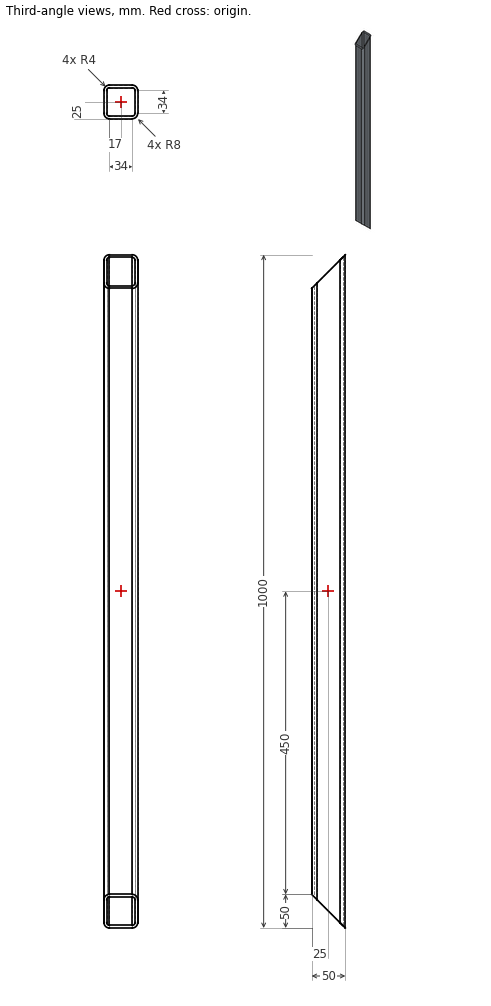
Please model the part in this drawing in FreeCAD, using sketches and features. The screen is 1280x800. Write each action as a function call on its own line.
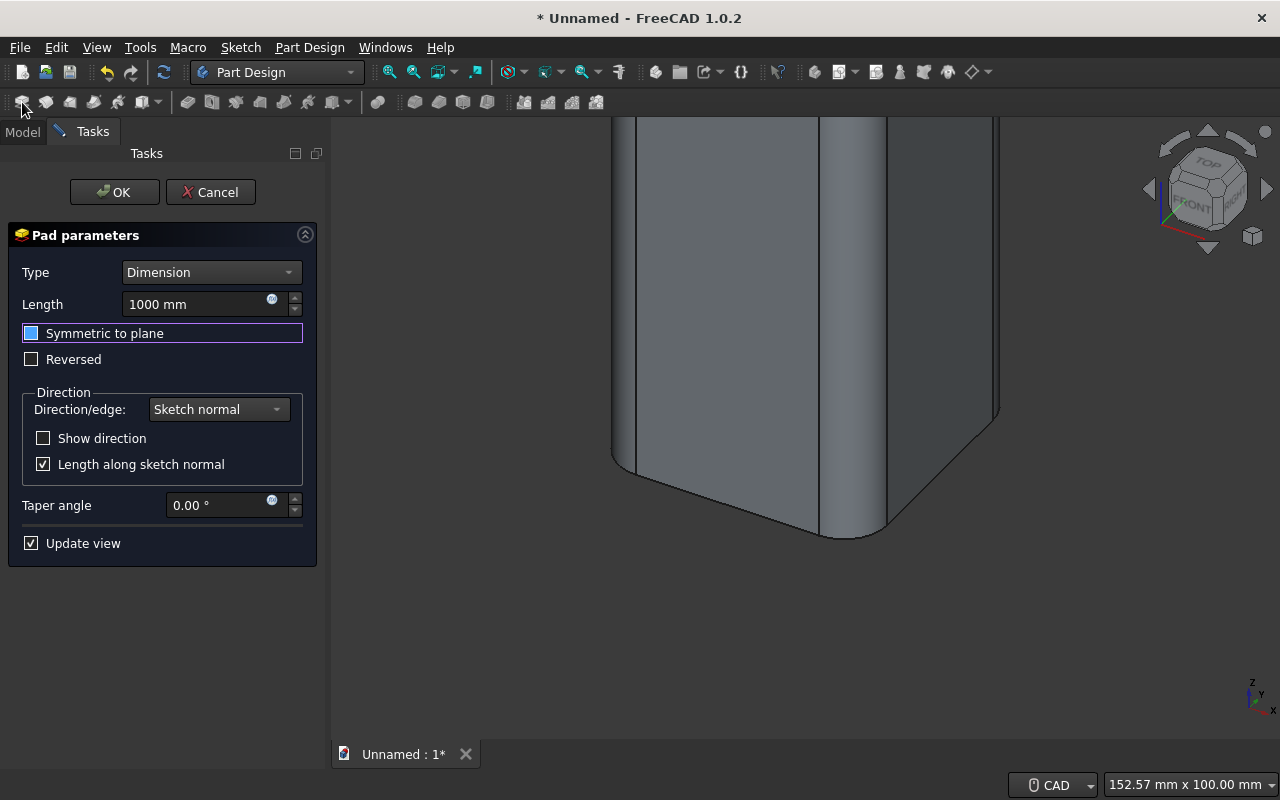
click(30, 333)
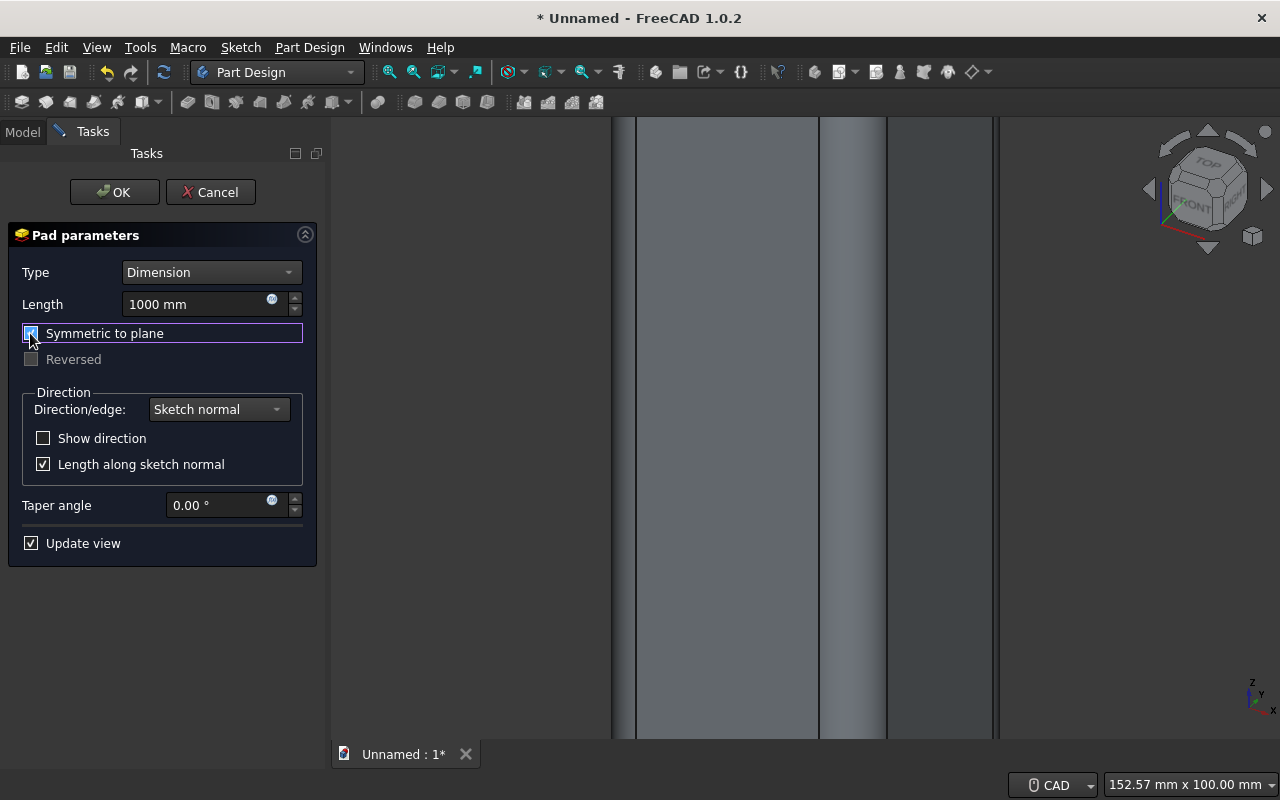
click(115, 192)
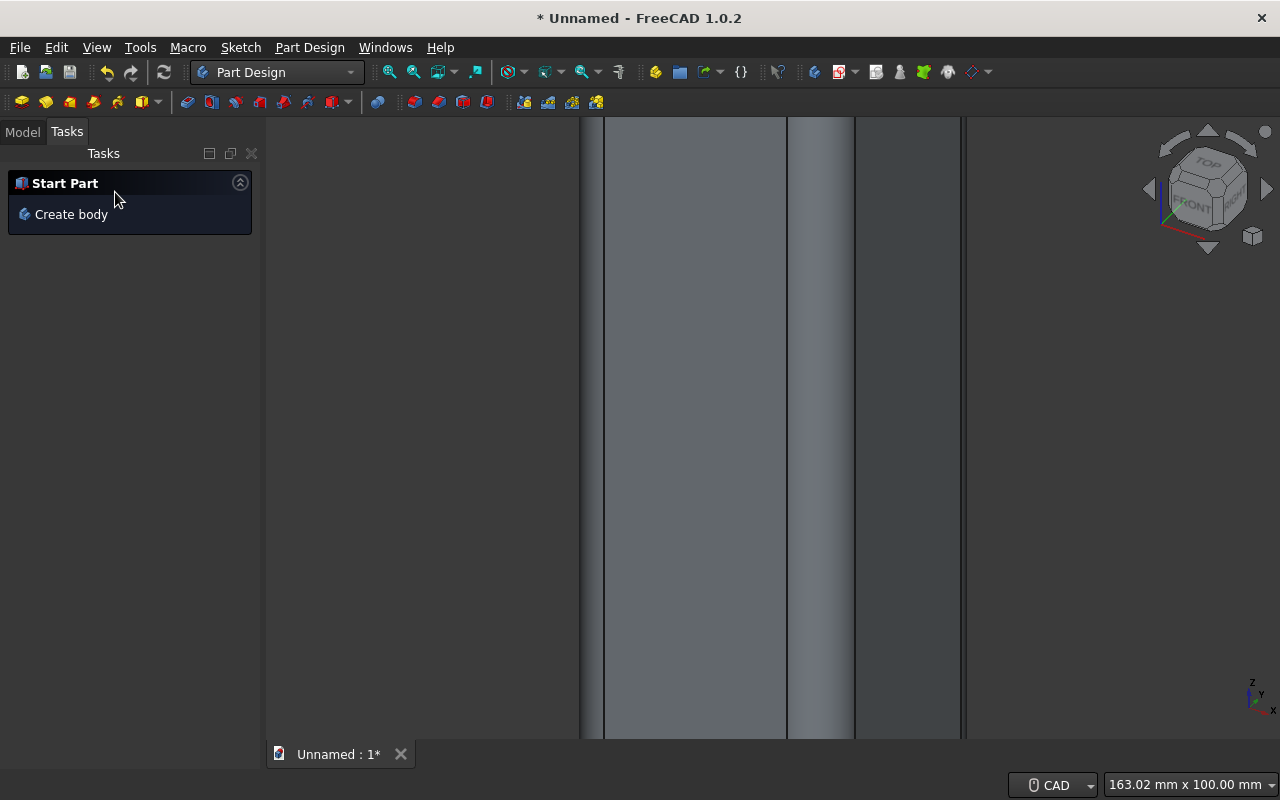
click(390, 72)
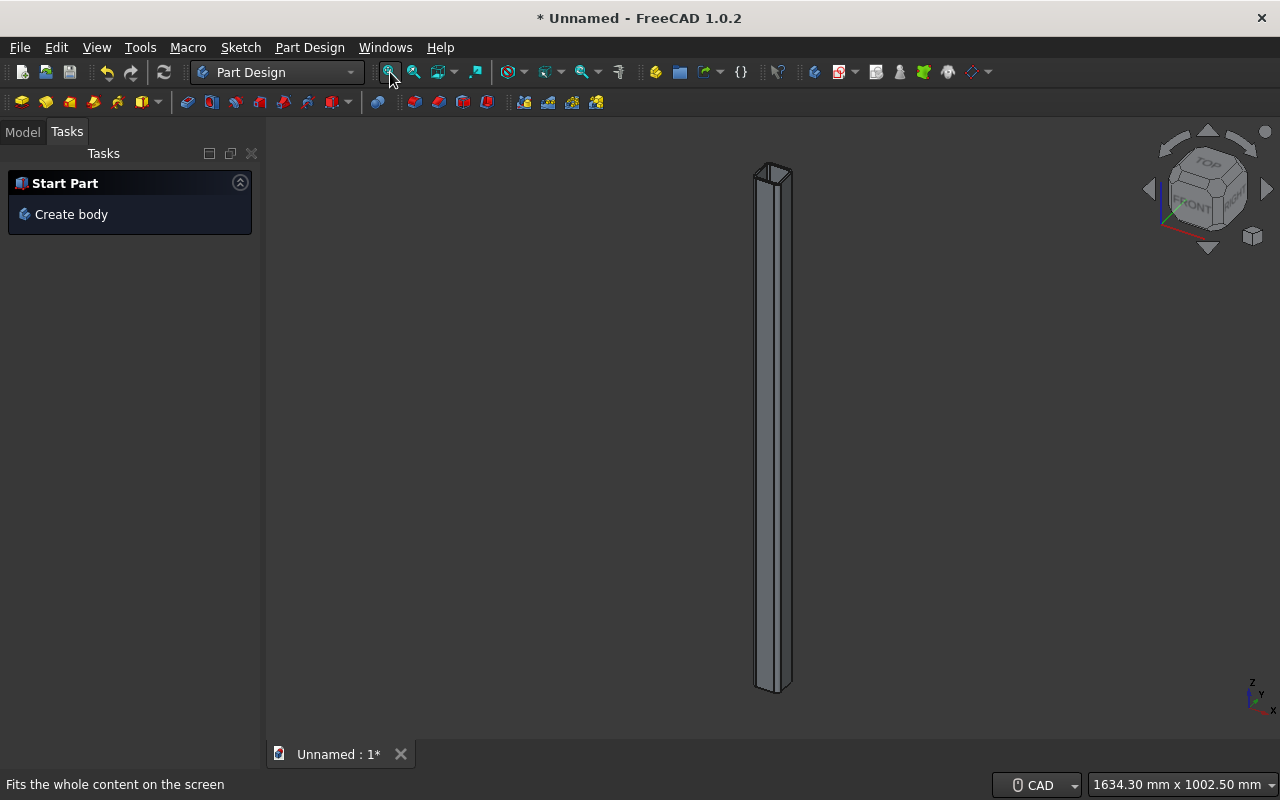
key(6)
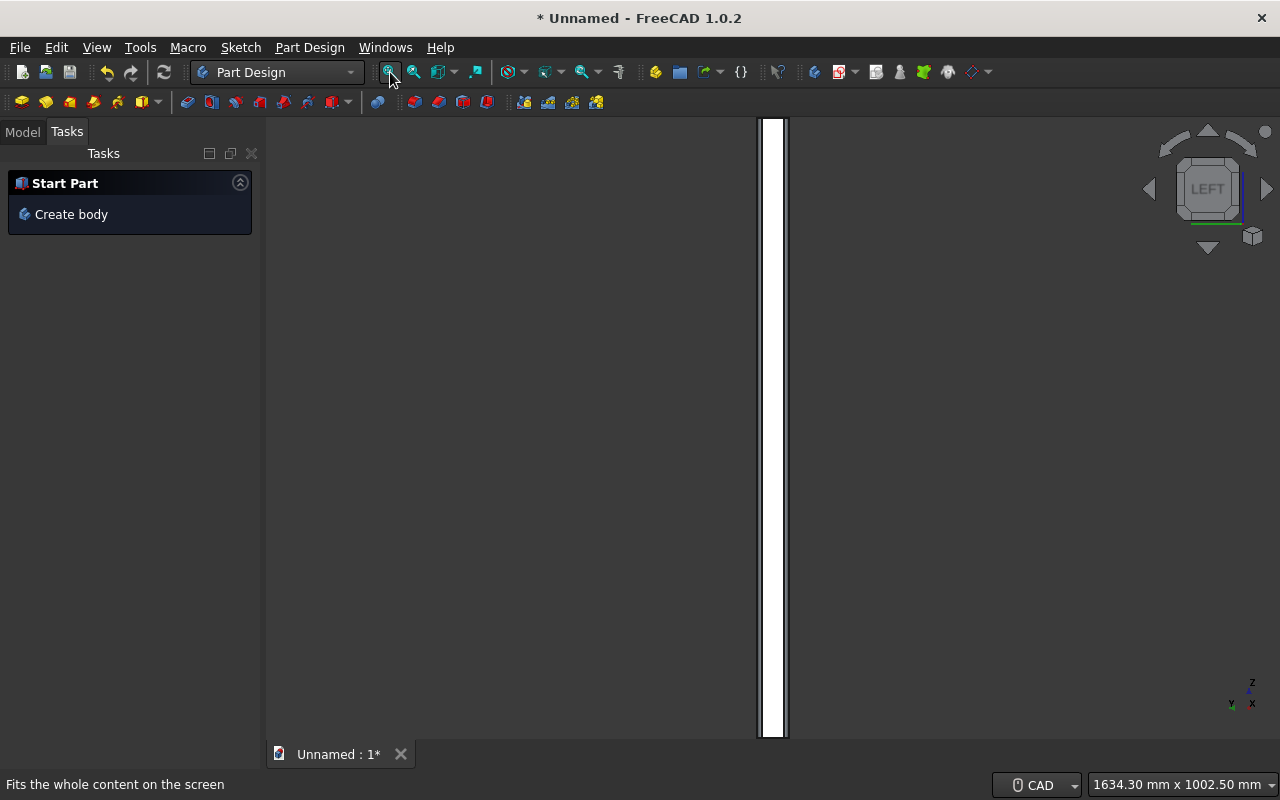
click(773, 161)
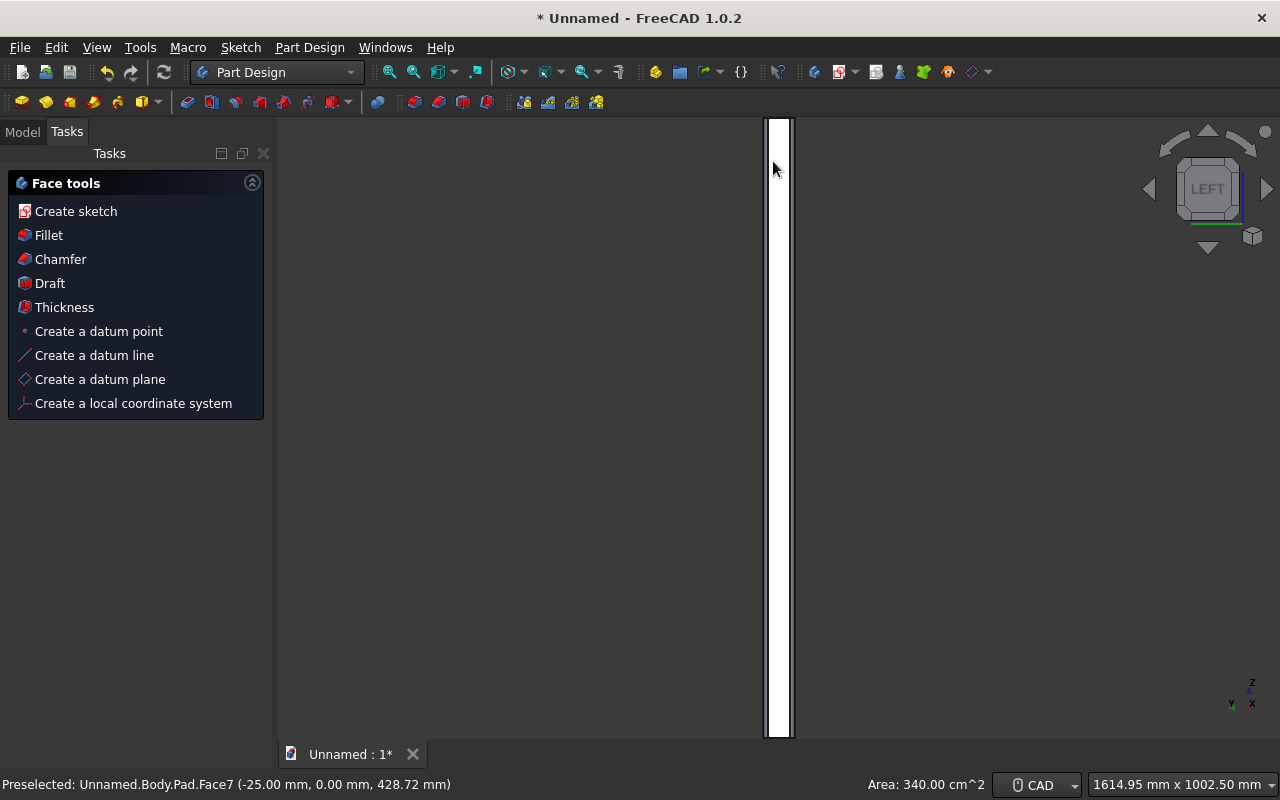
click(840, 72)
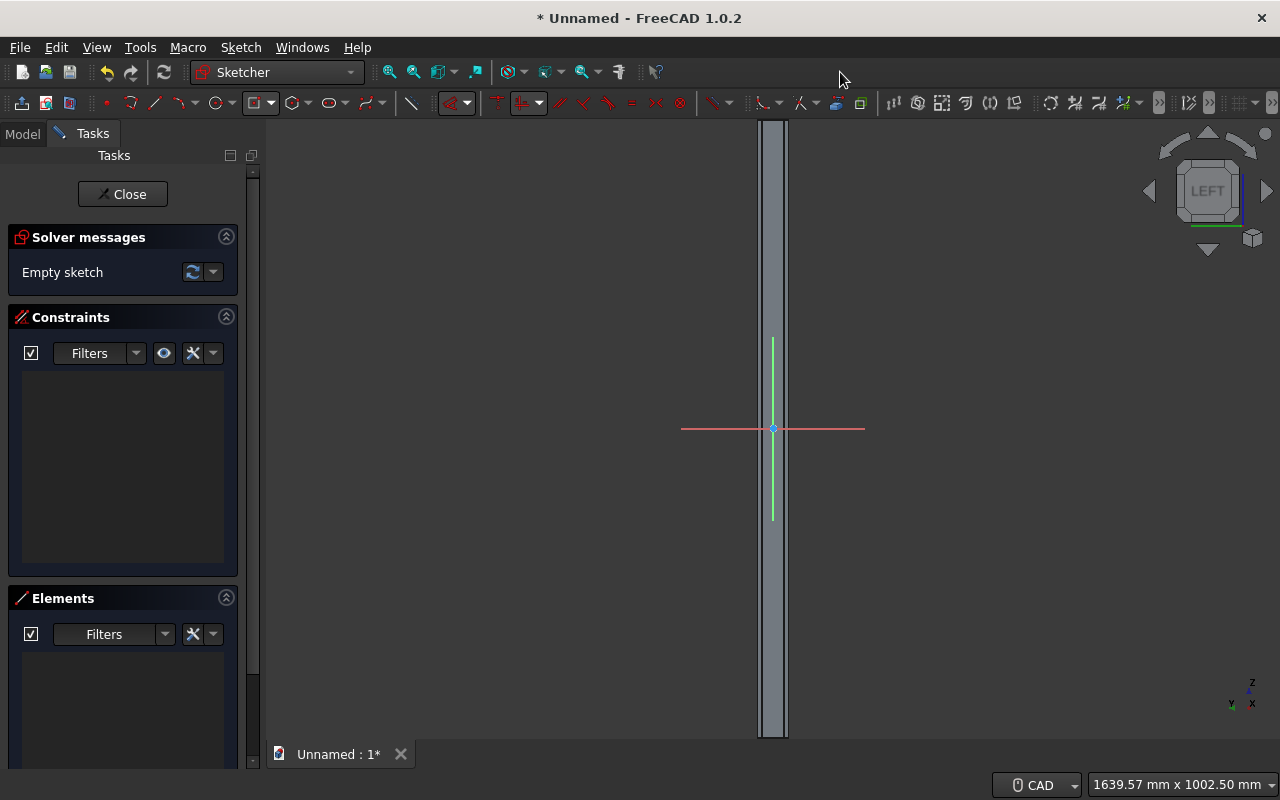
scroll(704, 429, down, 5)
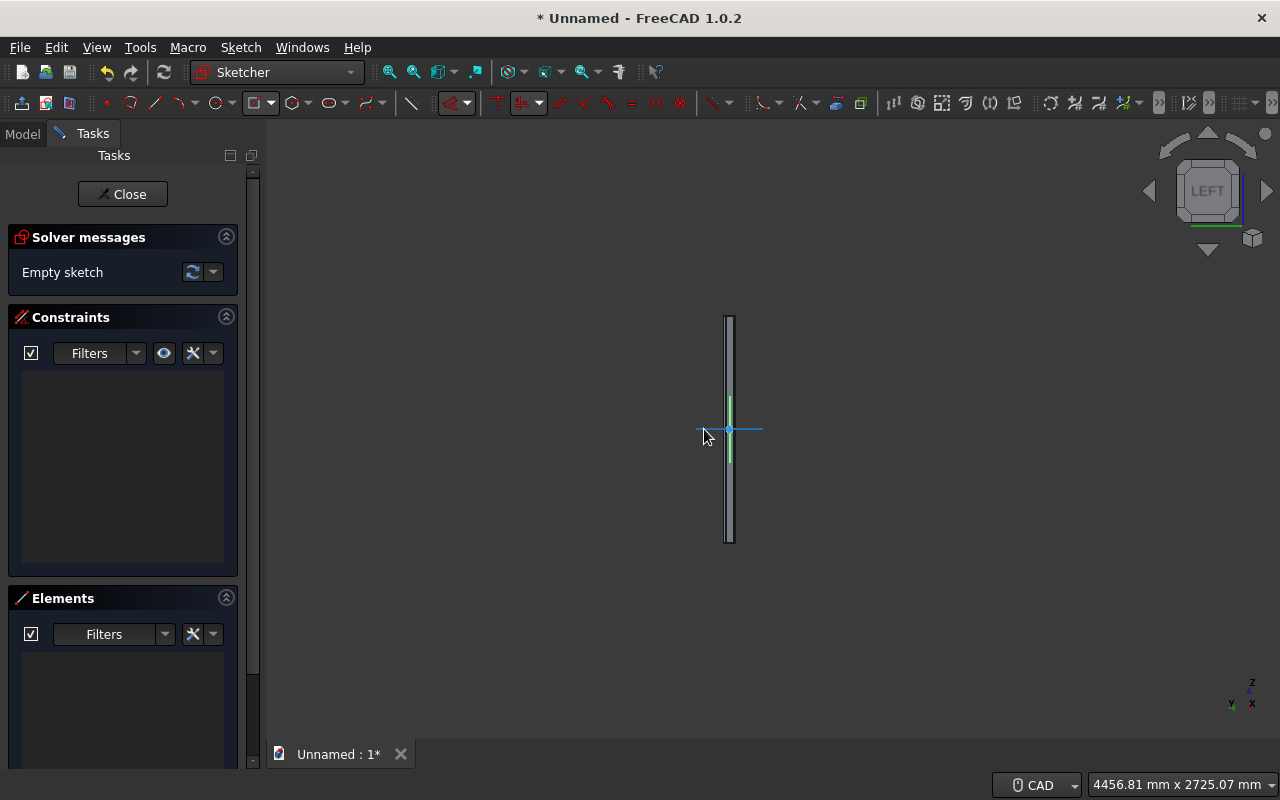
scroll(731, 543, up, 15)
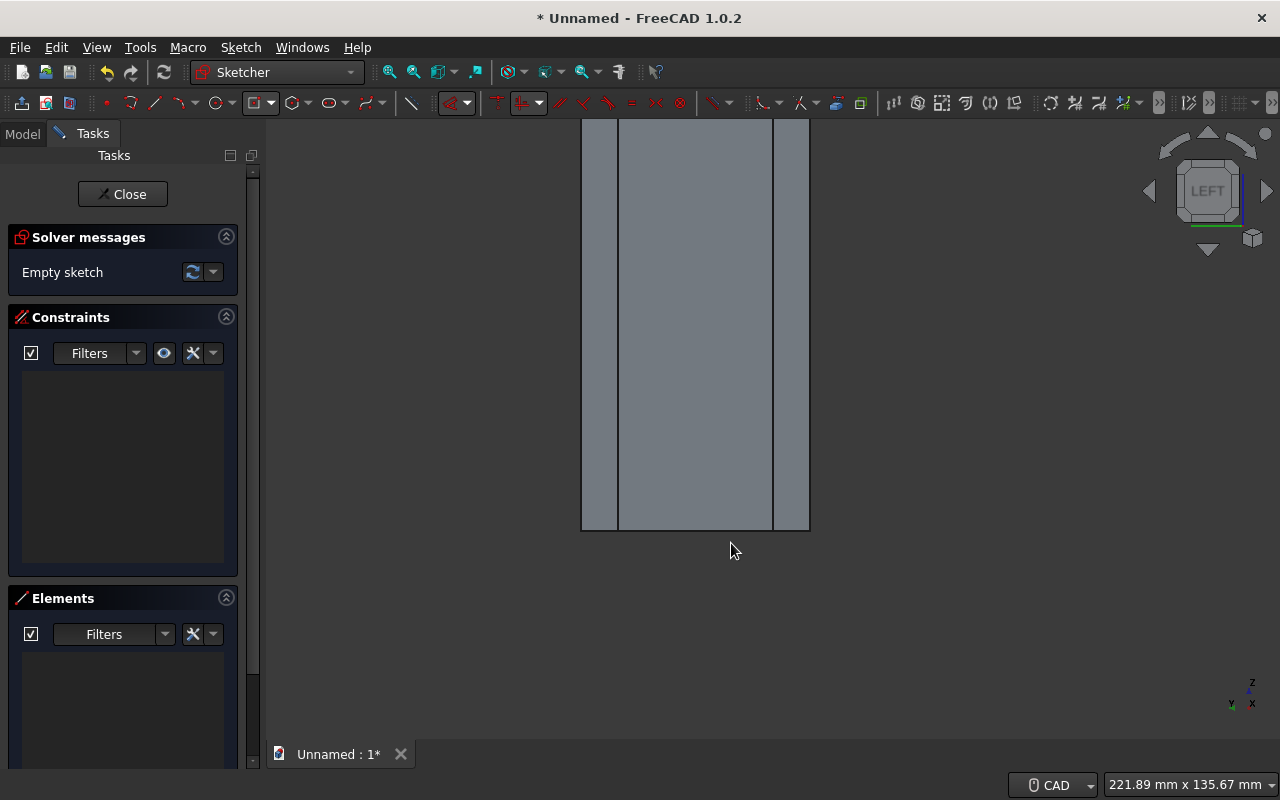
scroll(684, 403, up, 3)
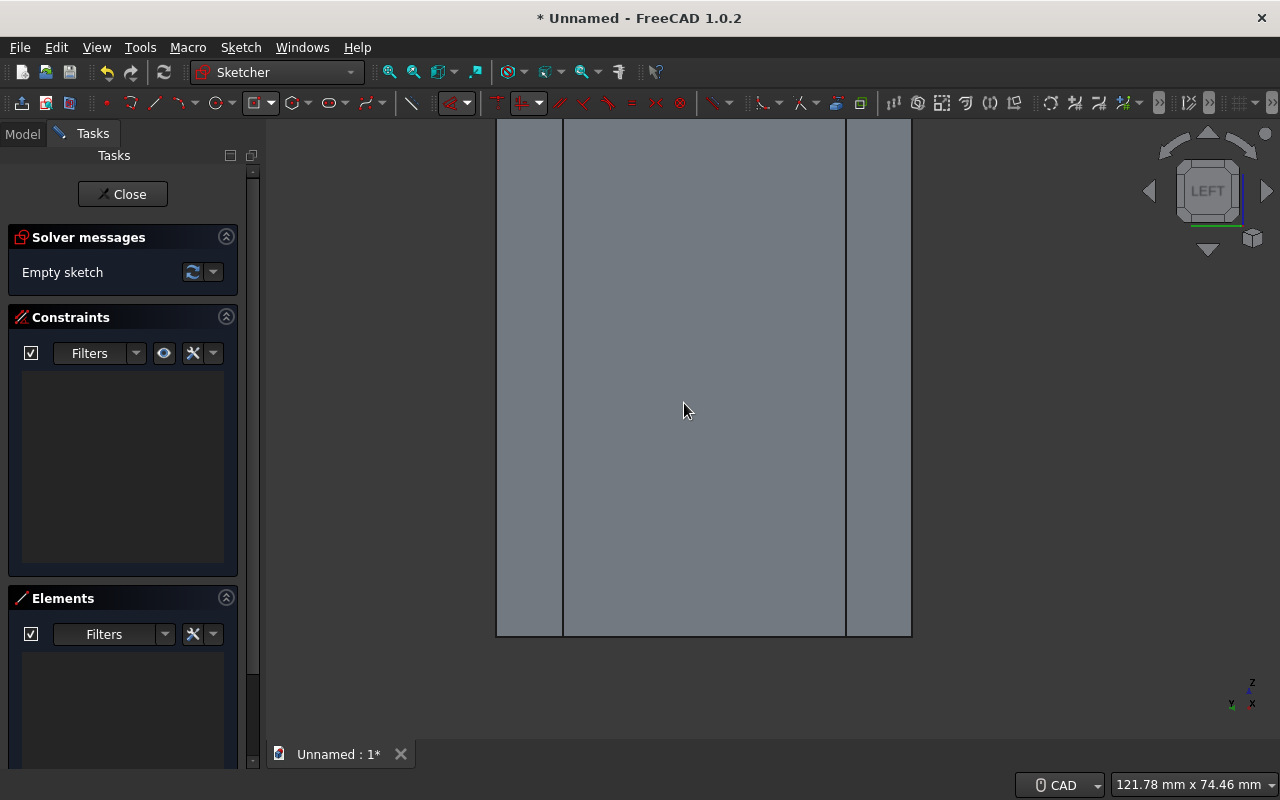
key(g)
key(m)